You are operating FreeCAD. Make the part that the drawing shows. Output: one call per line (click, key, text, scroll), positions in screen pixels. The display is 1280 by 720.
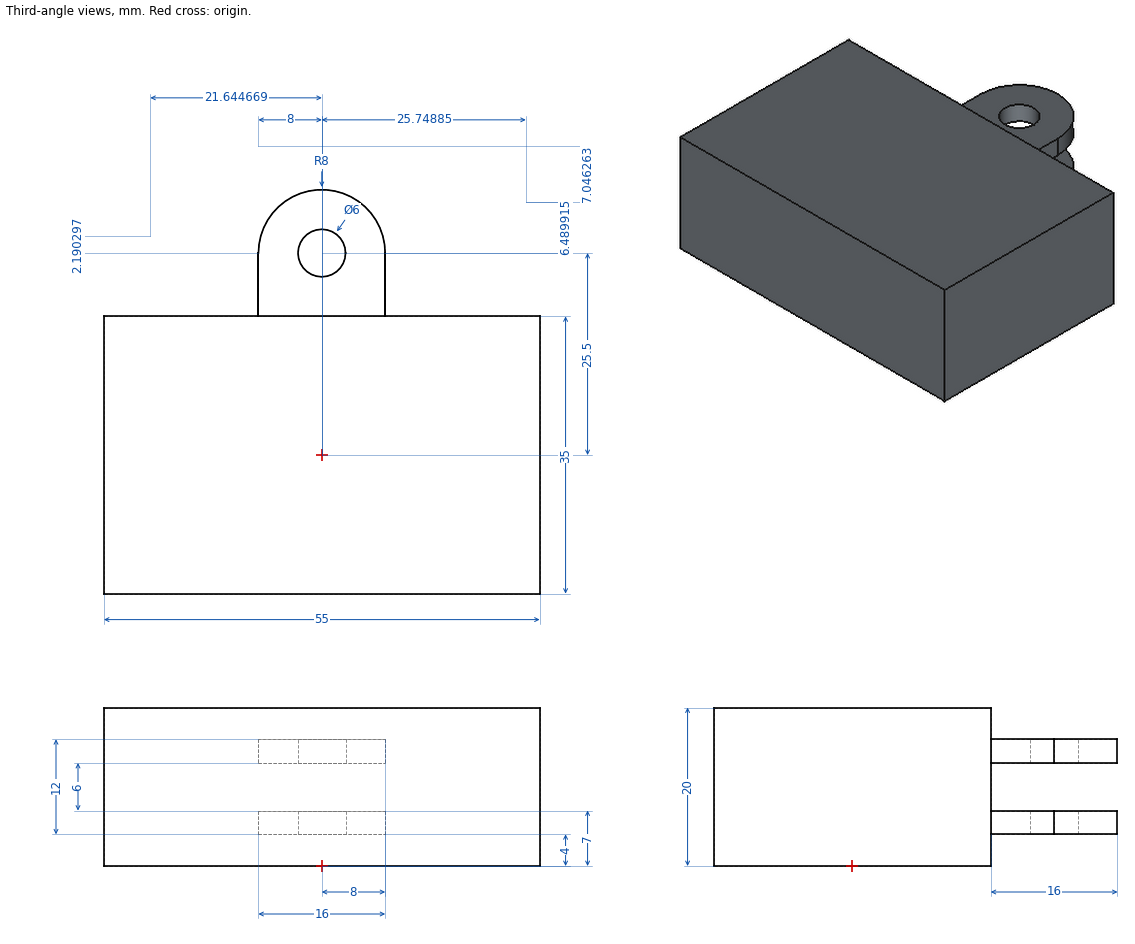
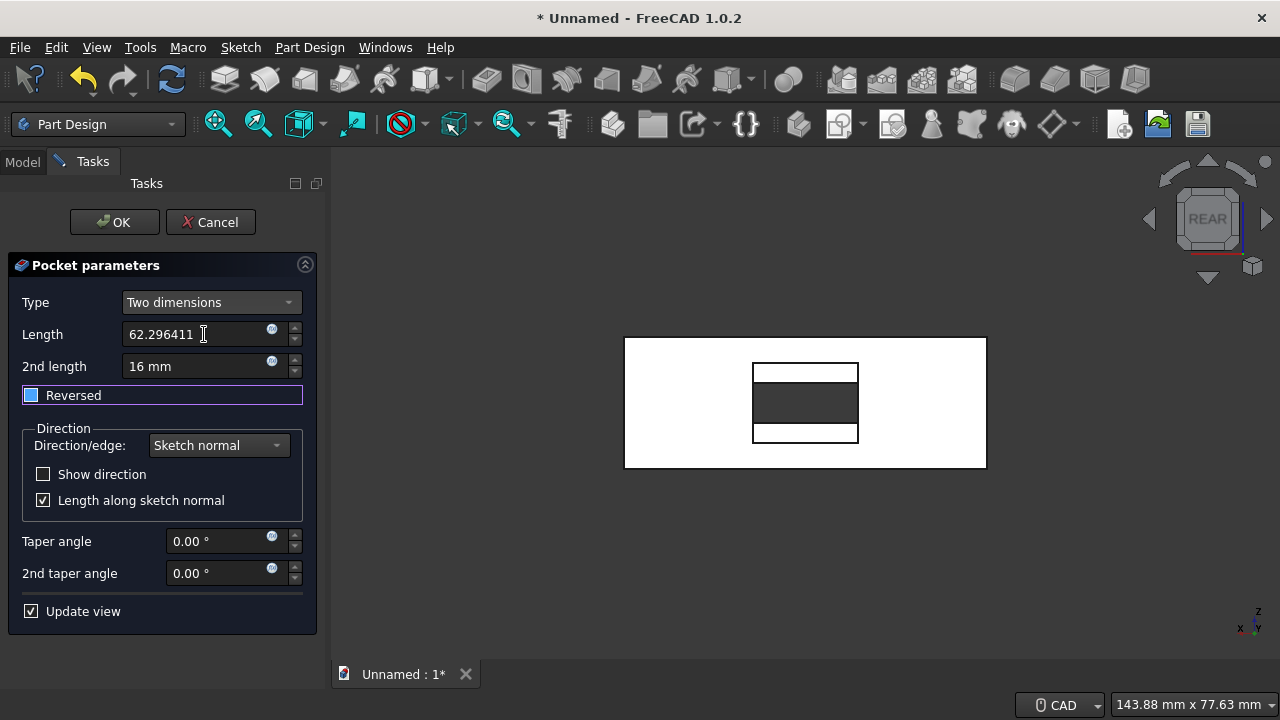
click(30, 395)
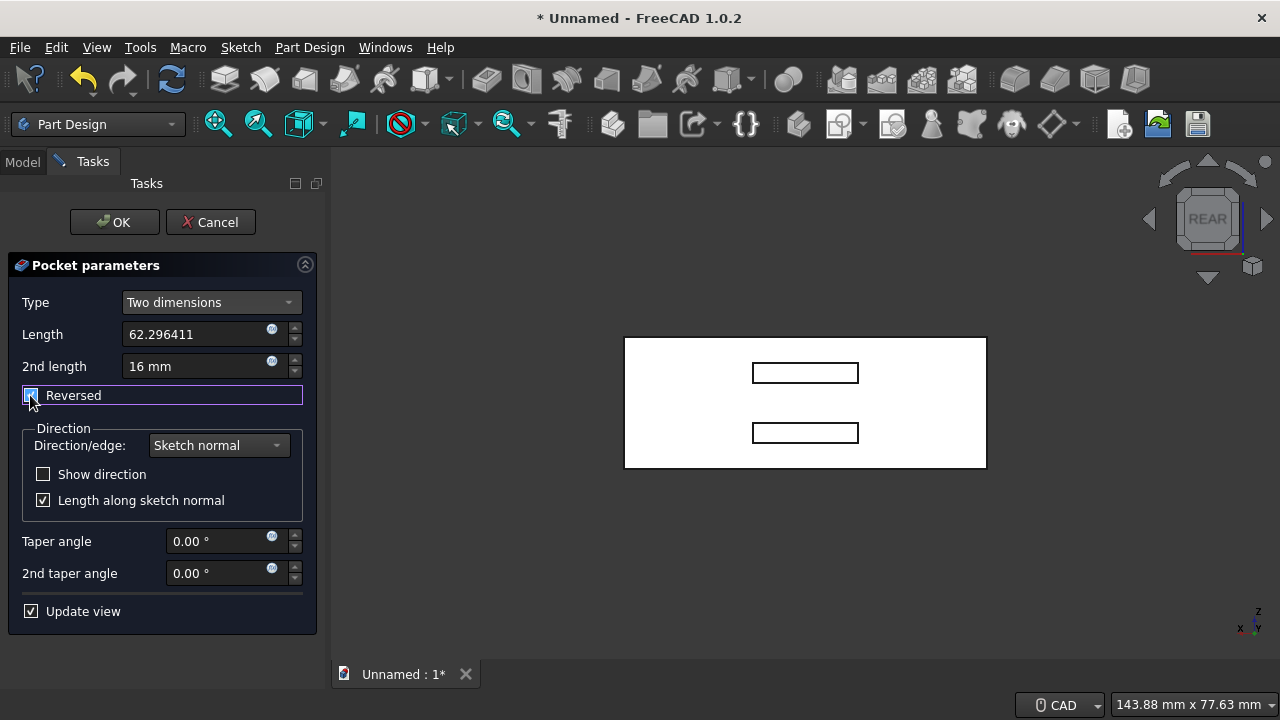
click(115, 222)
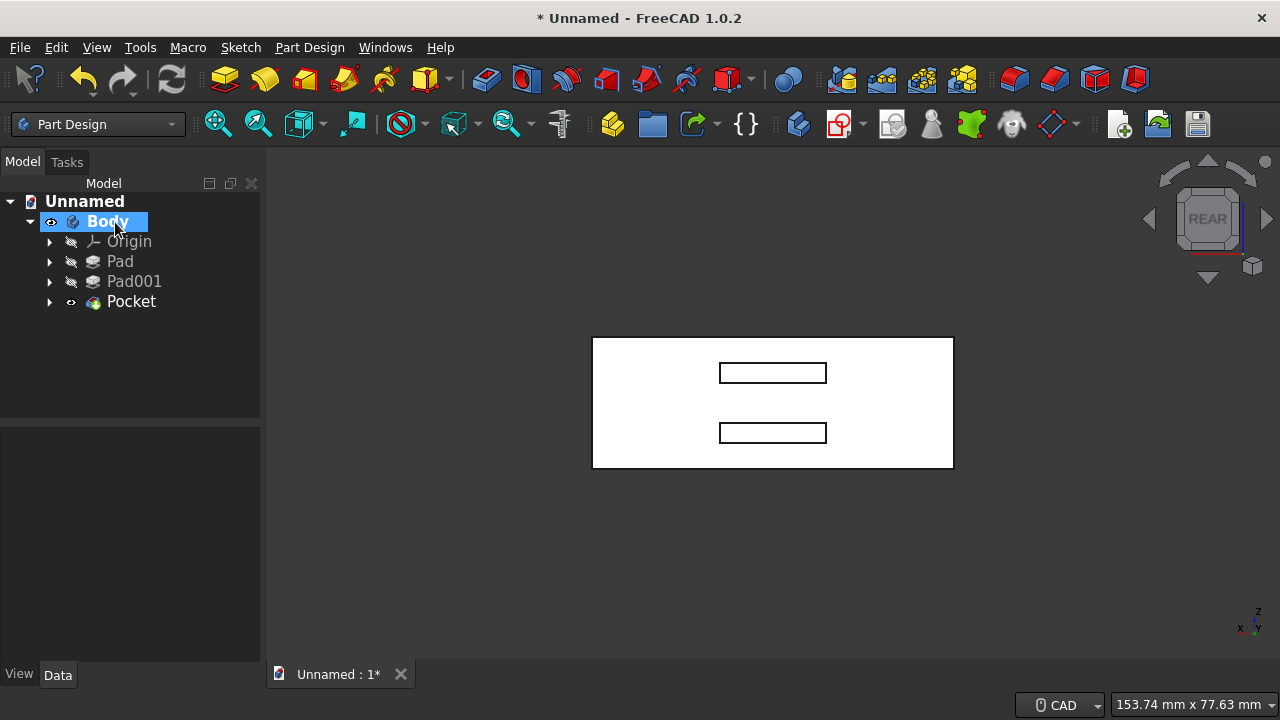
click(220, 124)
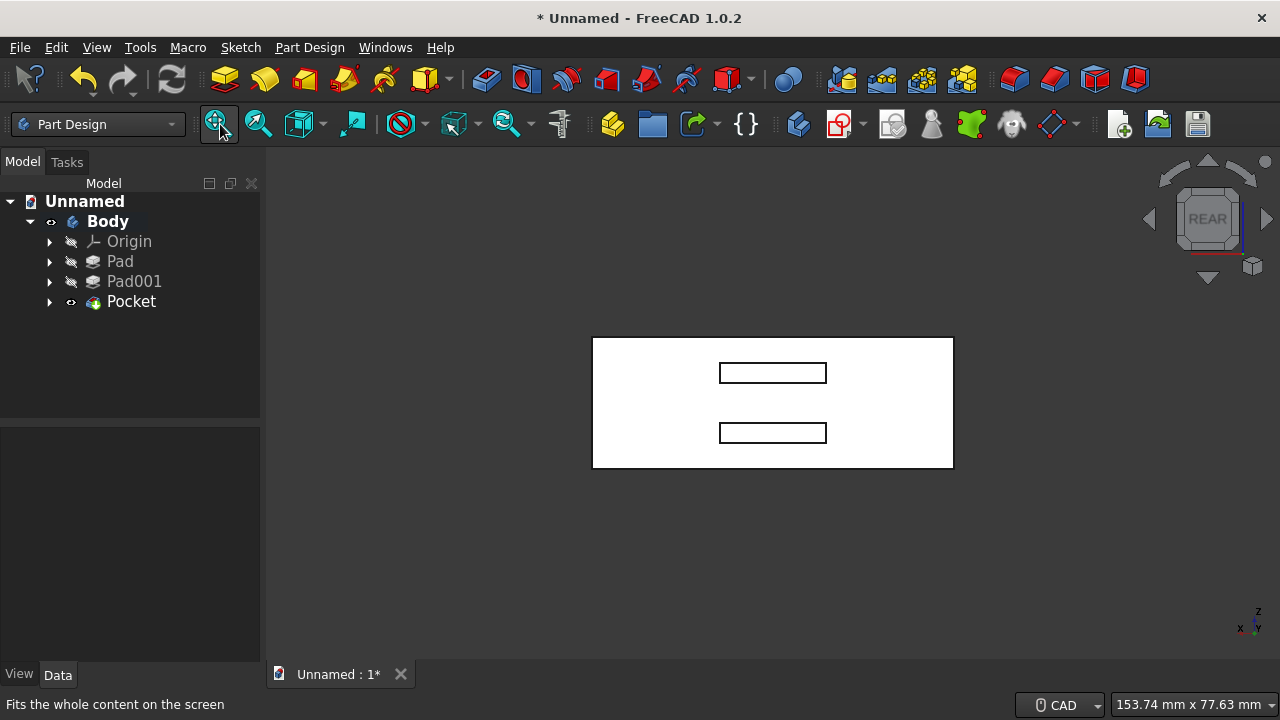
key(0)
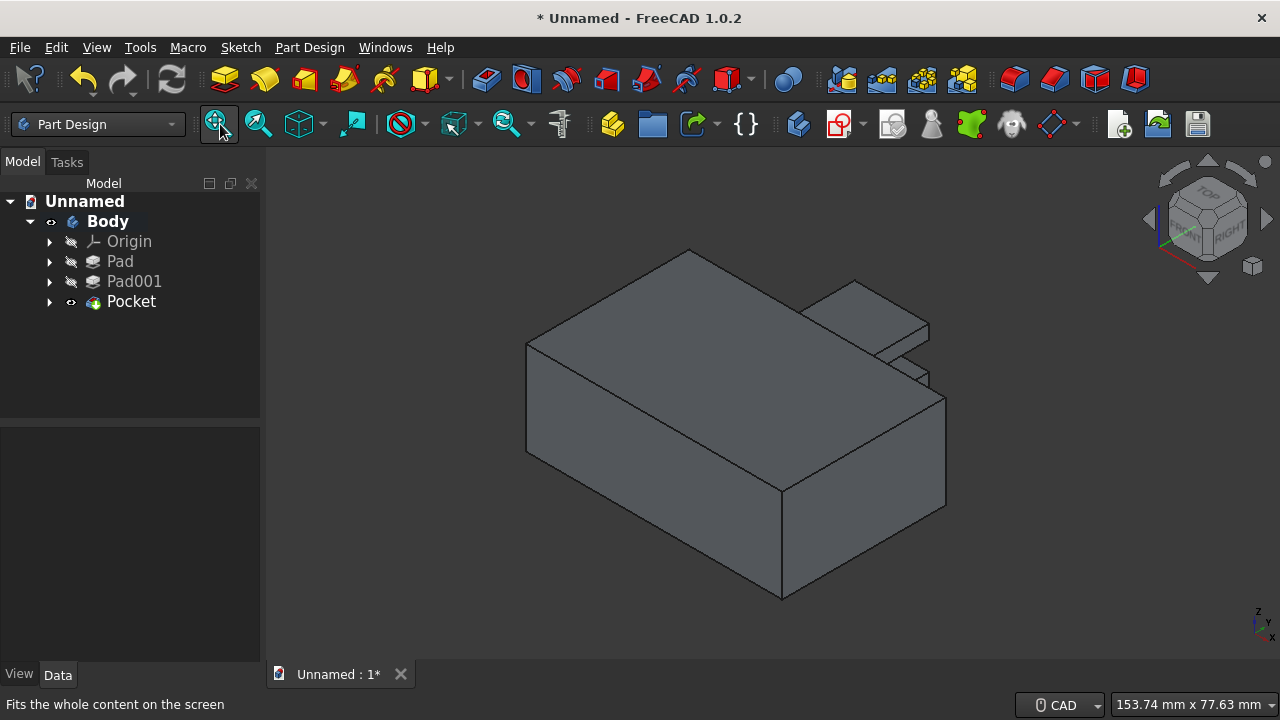
click(855, 323)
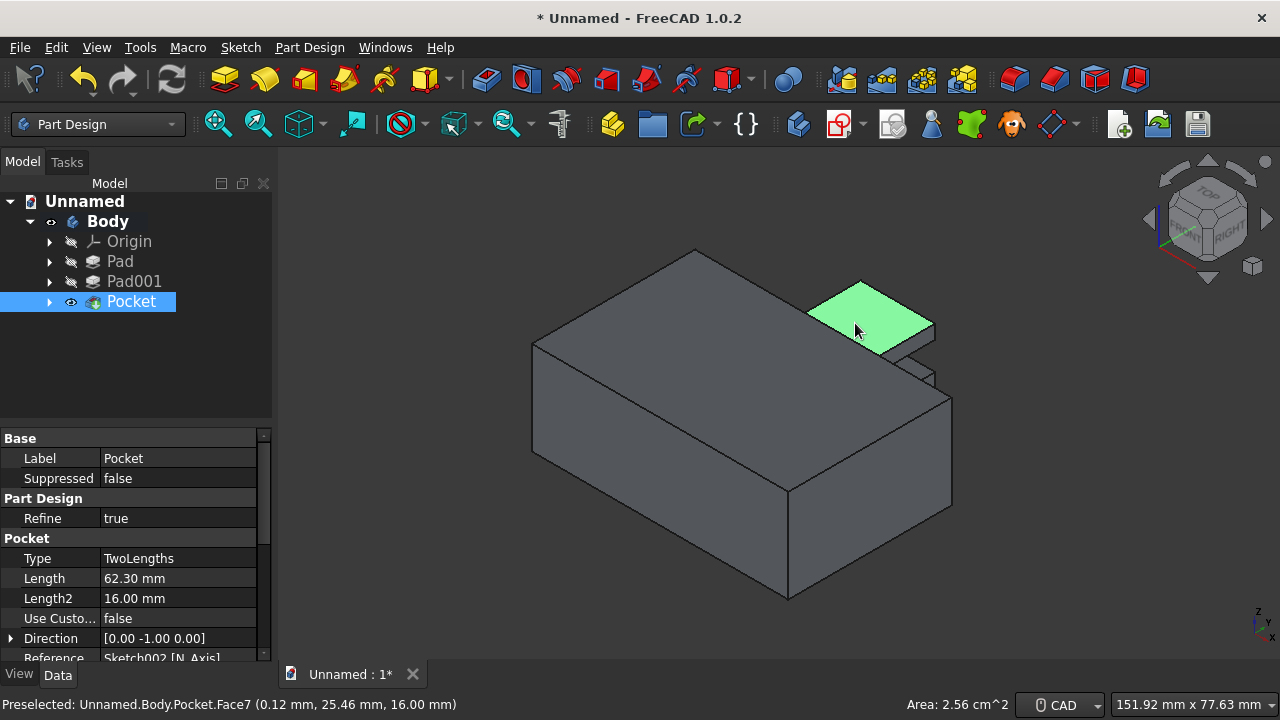
click(840, 124)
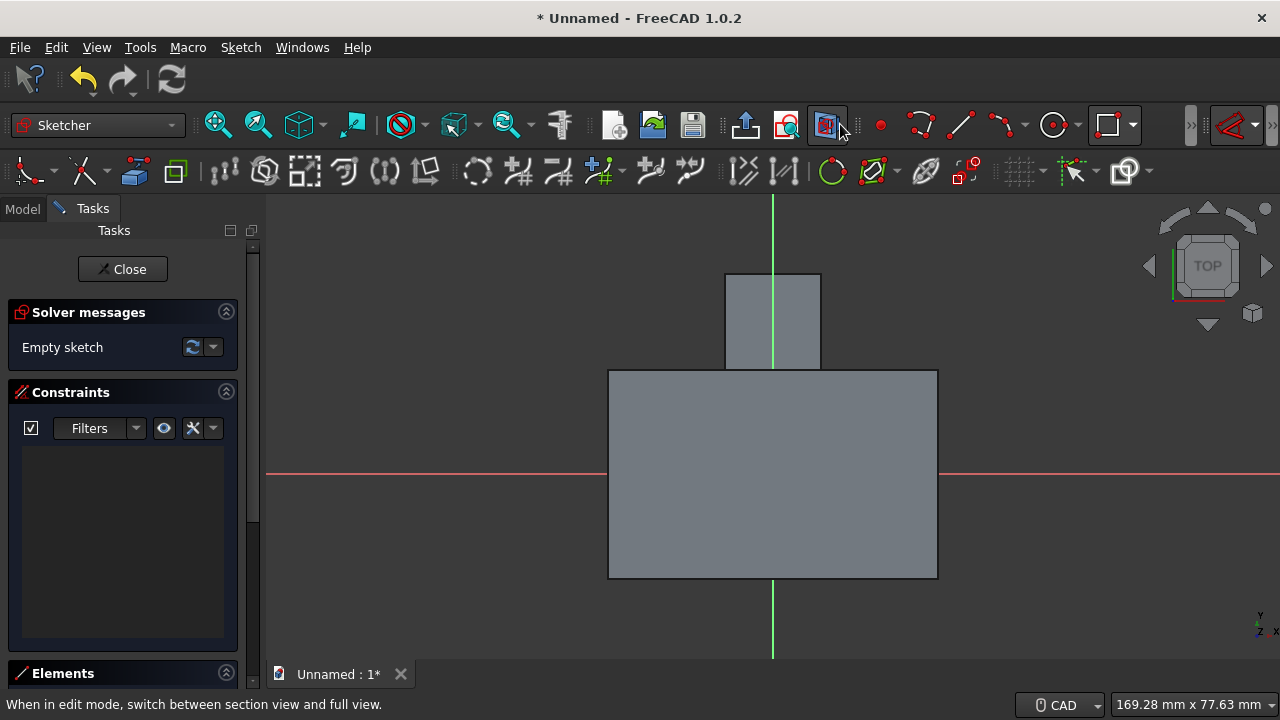
scroll(340, 631, down, 1)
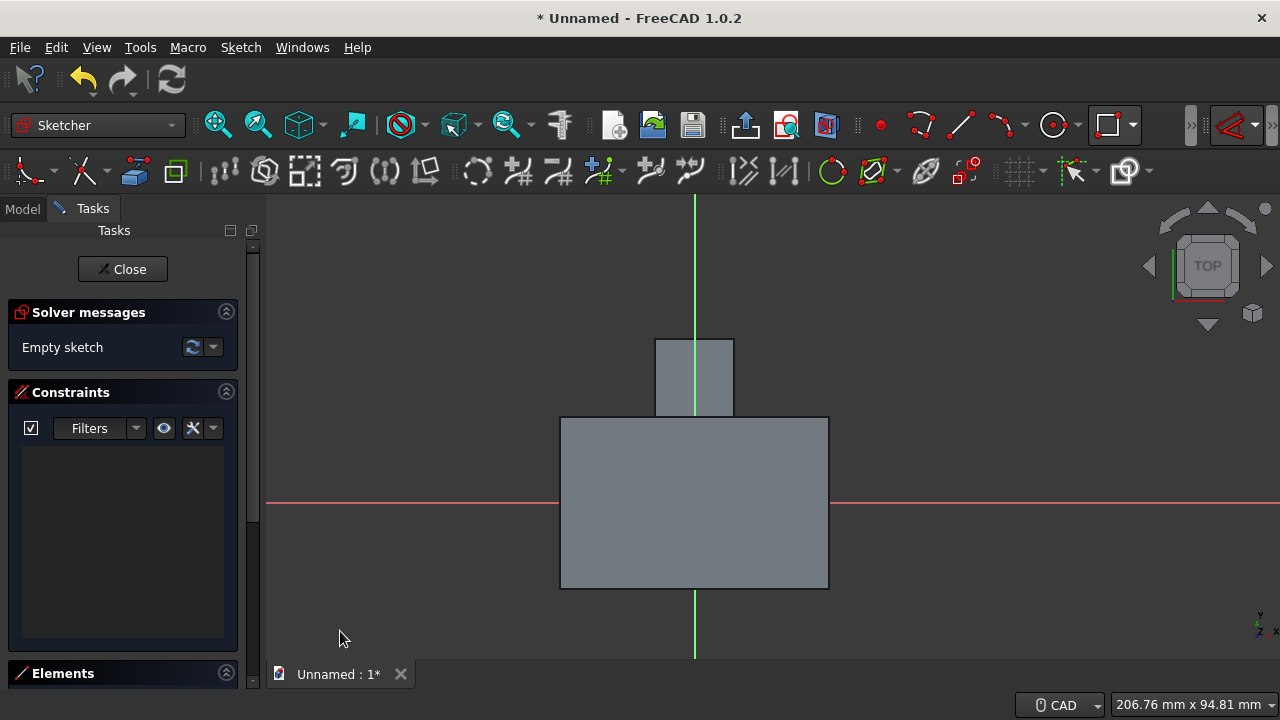
scroll(705, 368, up, 2)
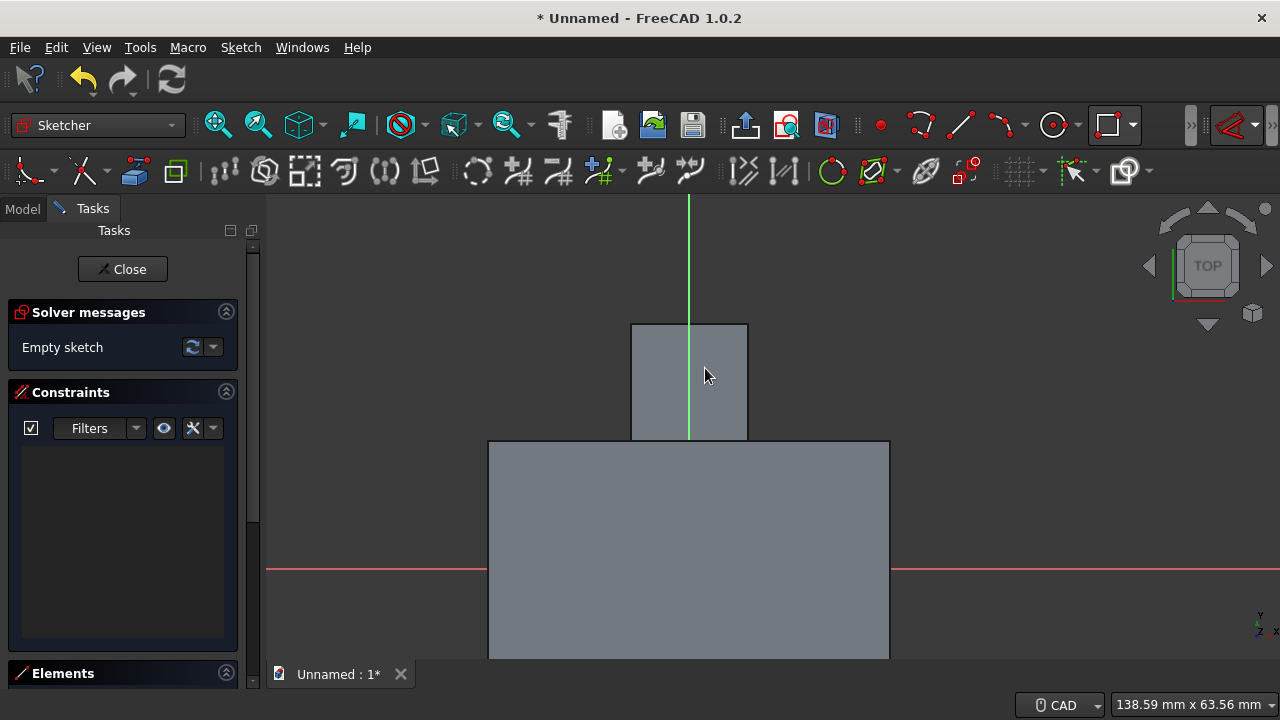
click(922, 126)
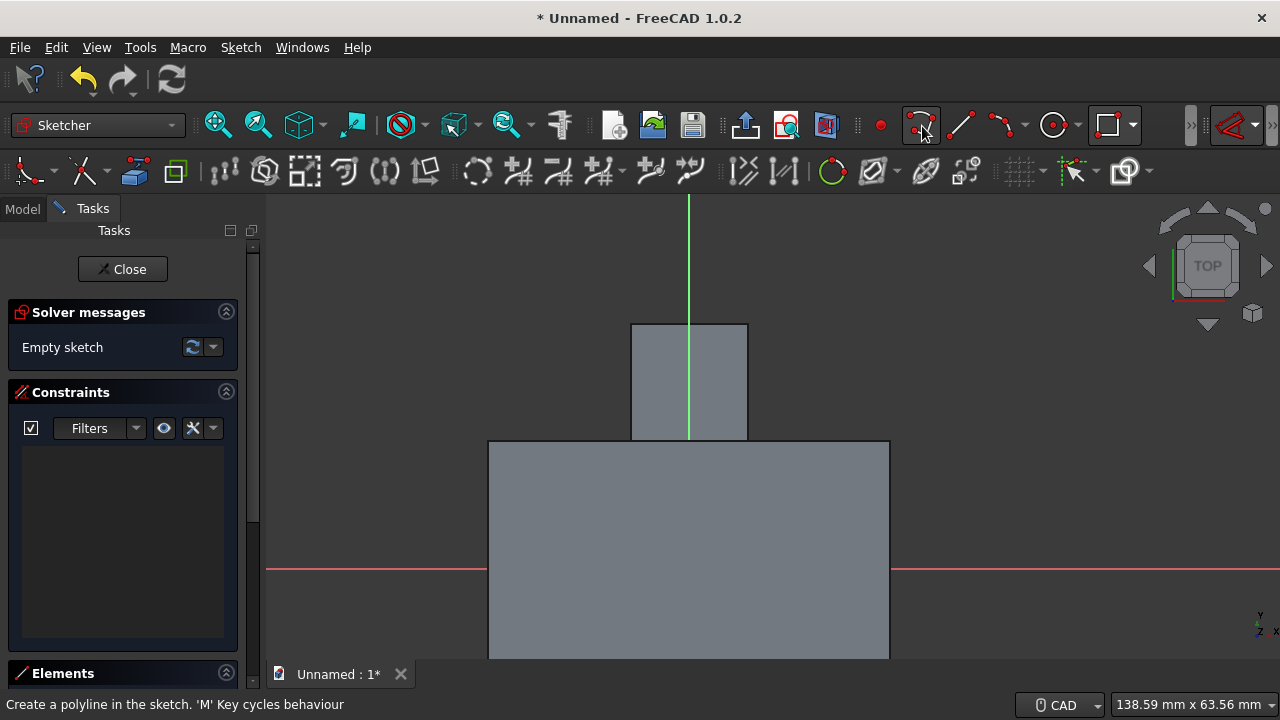
click(748, 383)
click(878, 335)
click(631, 284)
click(531, 367)
click(631, 383)
right_click(631, 383)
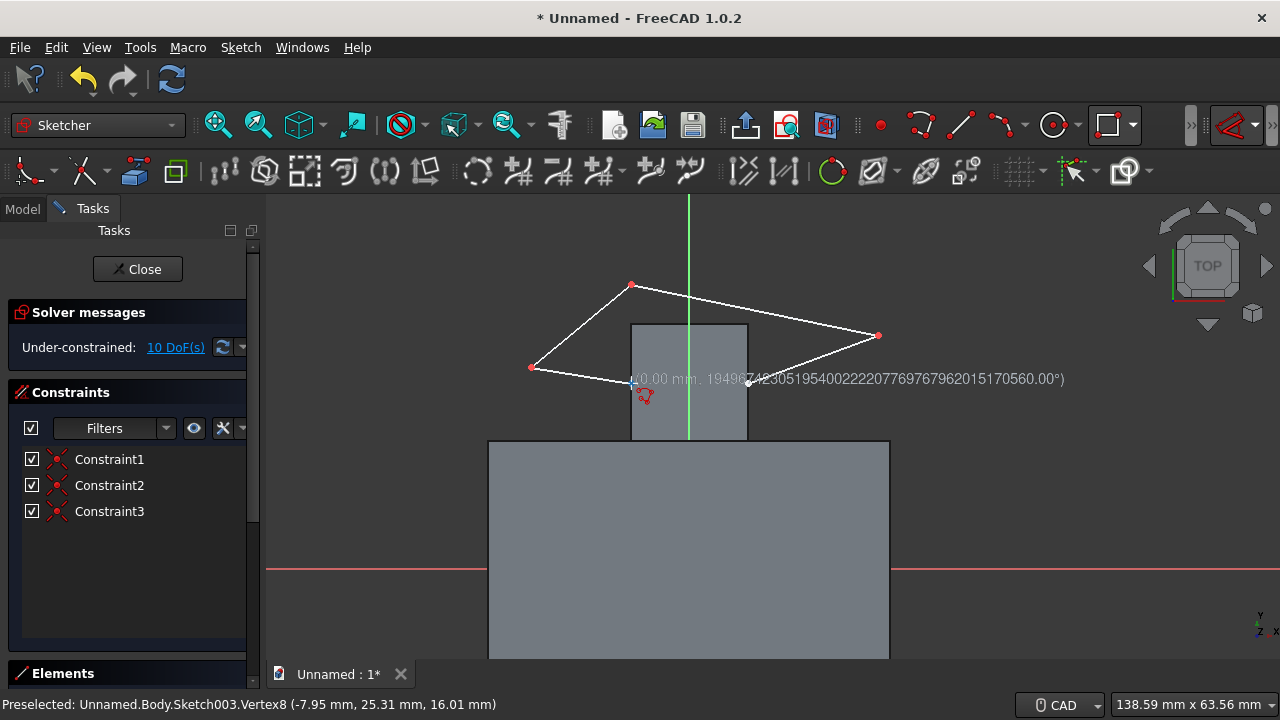
click(1002, 126)